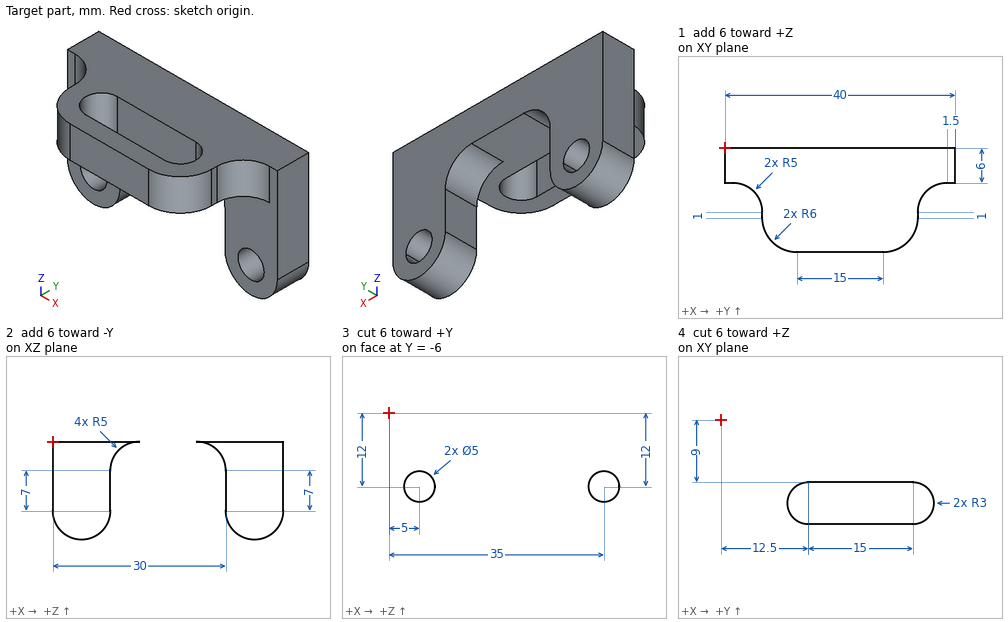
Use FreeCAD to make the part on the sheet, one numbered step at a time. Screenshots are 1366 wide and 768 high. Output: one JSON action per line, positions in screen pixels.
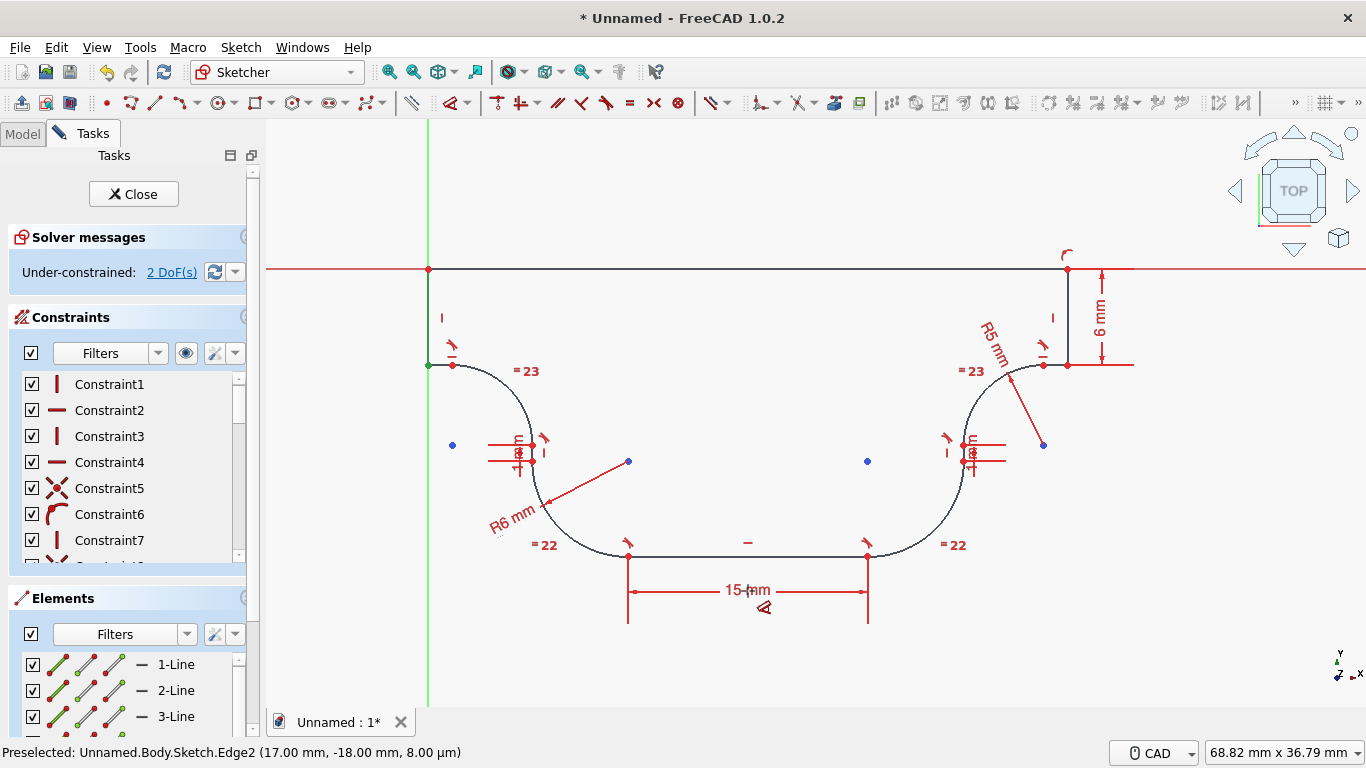
{"action": "left_click", "coordinate": [876, 269]}
{"action": "left_click", "coordinate": [748, 235]}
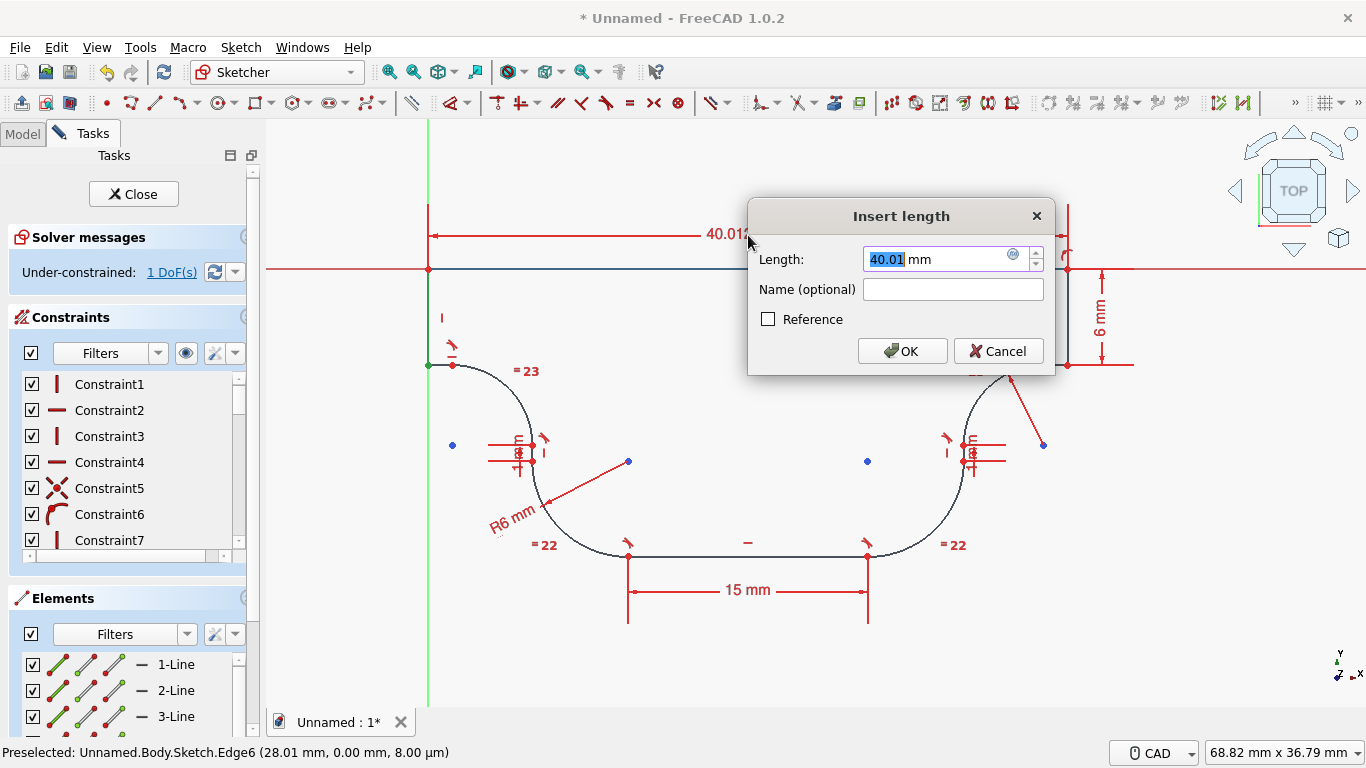
{"action": "type", "text": "40"}
{"action": "key", "text": "Return"}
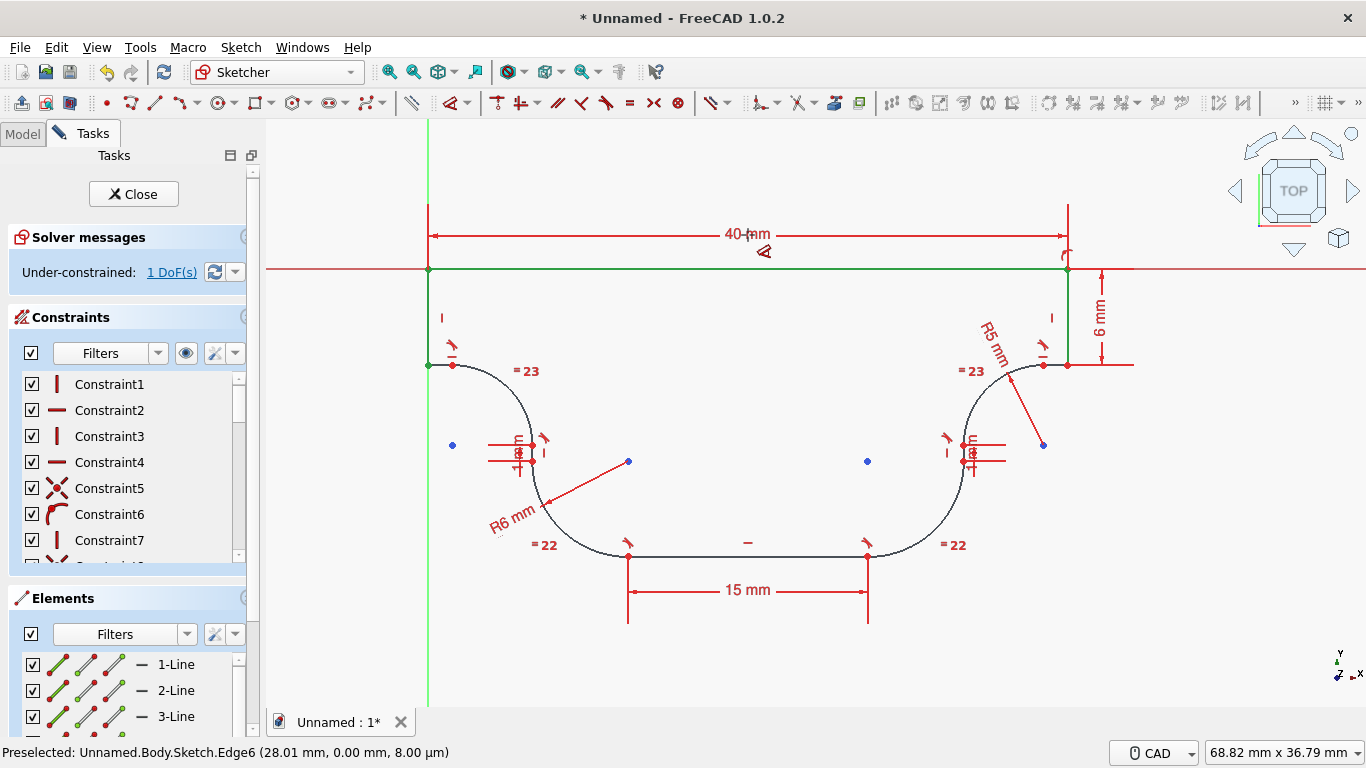
{"action": "scroll", "coordinate": [1053, 365], "scroll_direction": "up", "scroll_amount": 3}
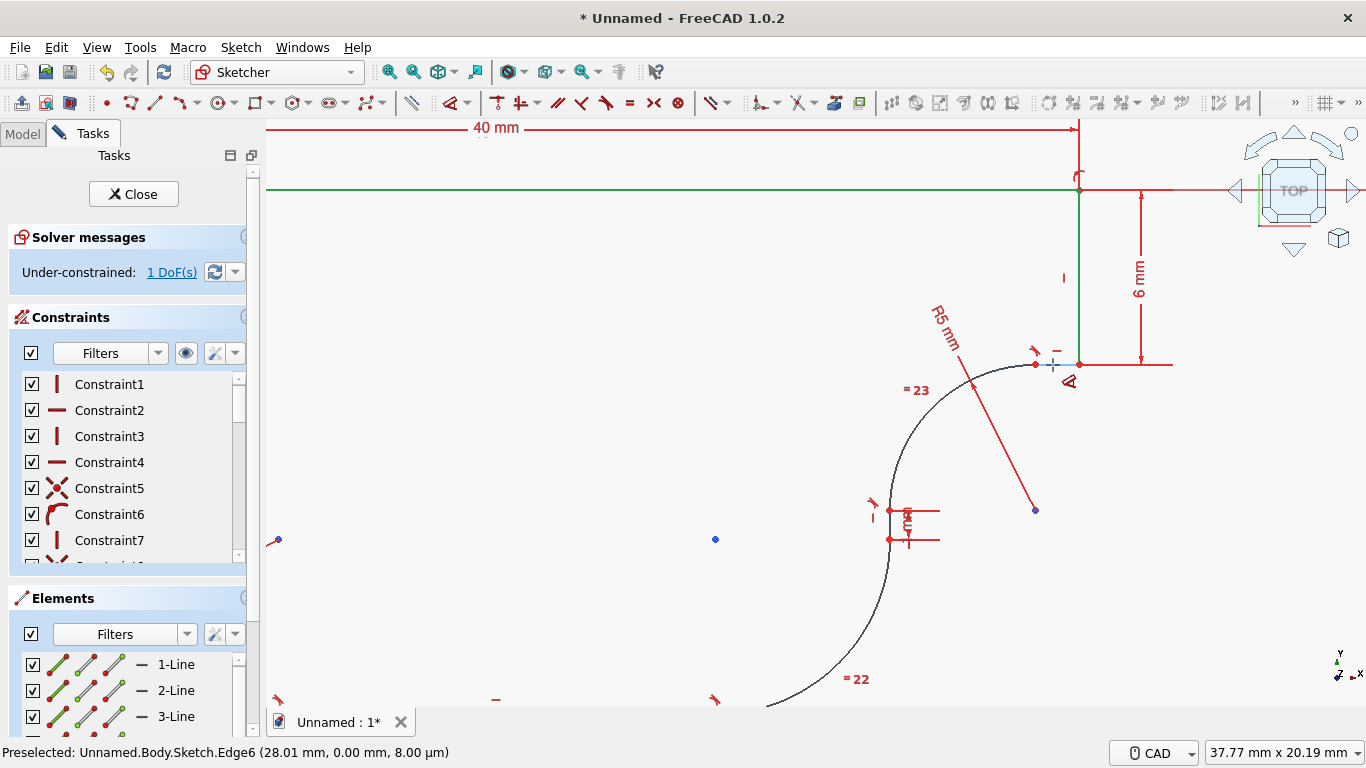
{"action": "left_click", "coordinate": [1053, 365]}
{"action": "left_click", "coordinate": [1057, 331]}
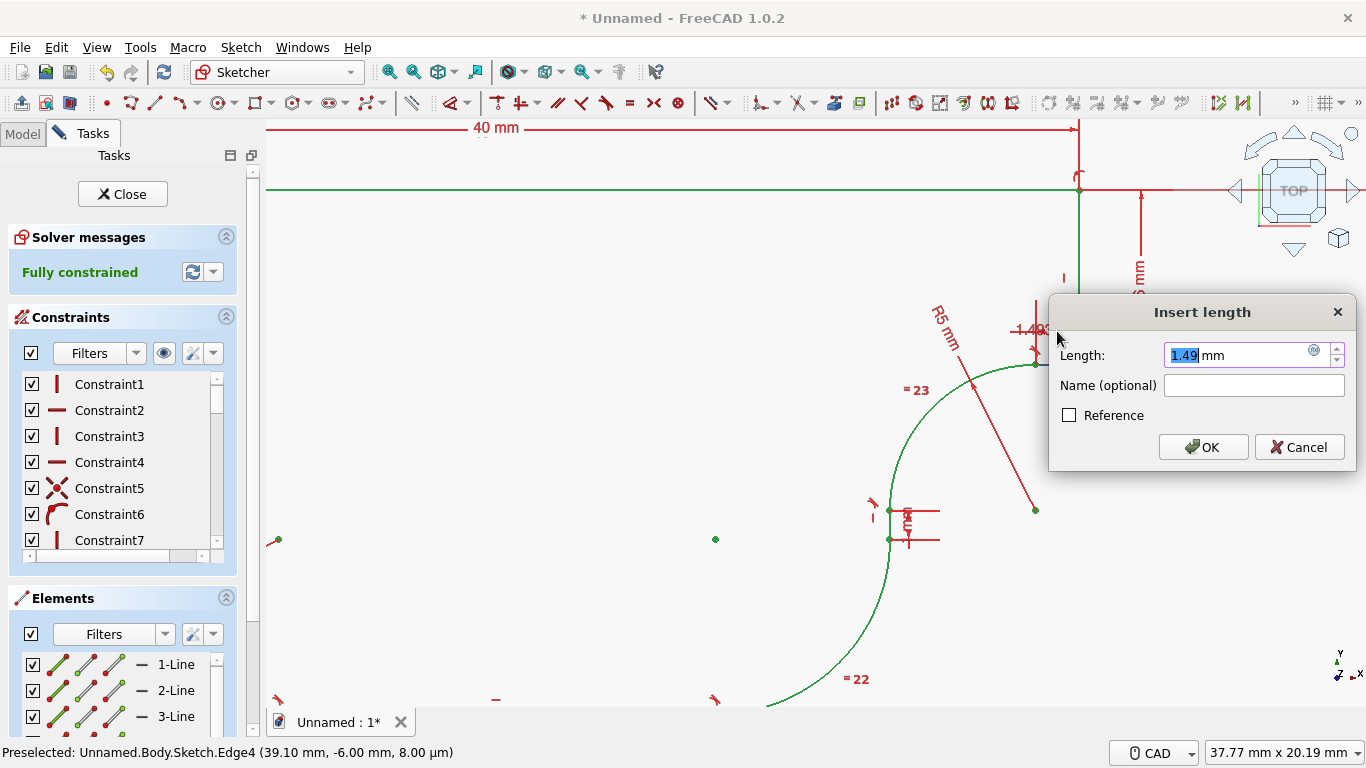
{"action": "type", "text": "1.5"}
{"action": "key", "text": "Return"}
{"action": "key", "text": "Escape"}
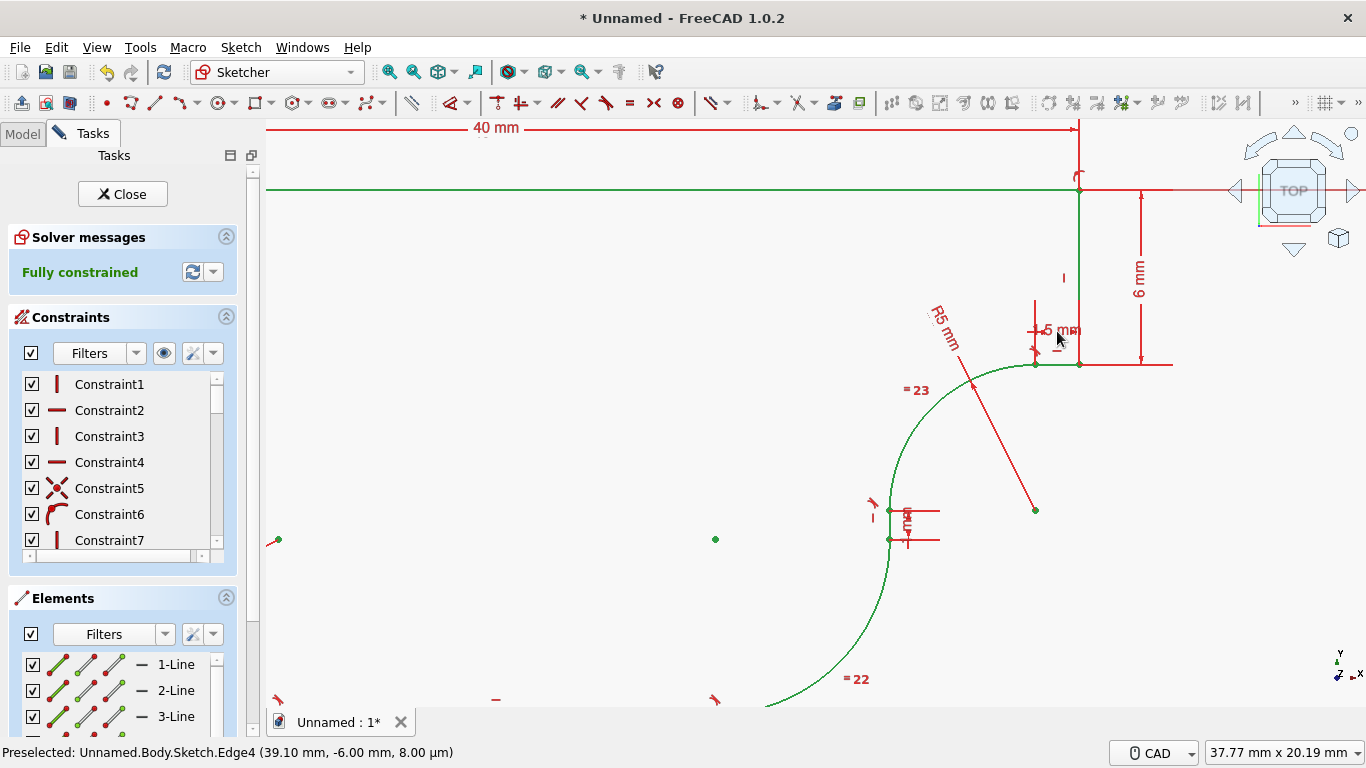
{"action": "left_click", "coordinate": [123, 194]}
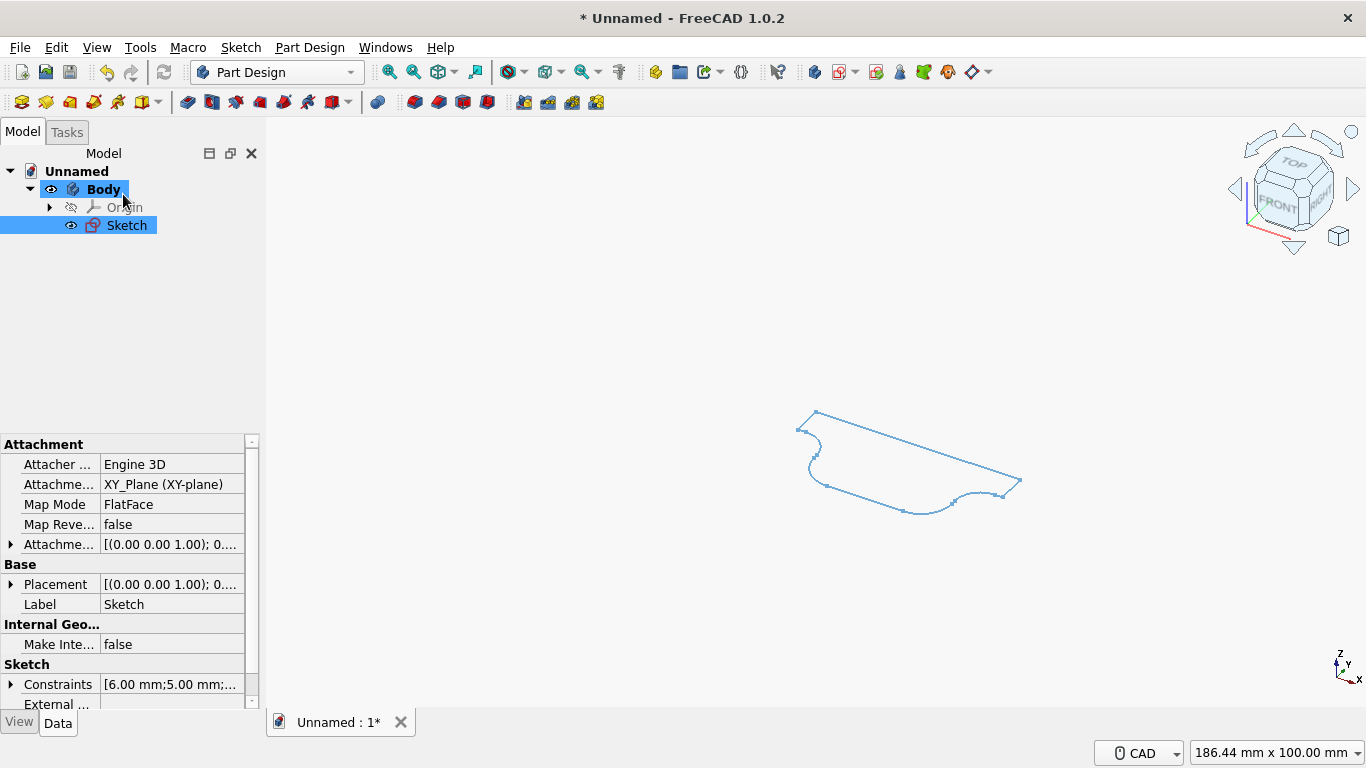
{"action": "left_click", "coordinate": [22, 102]}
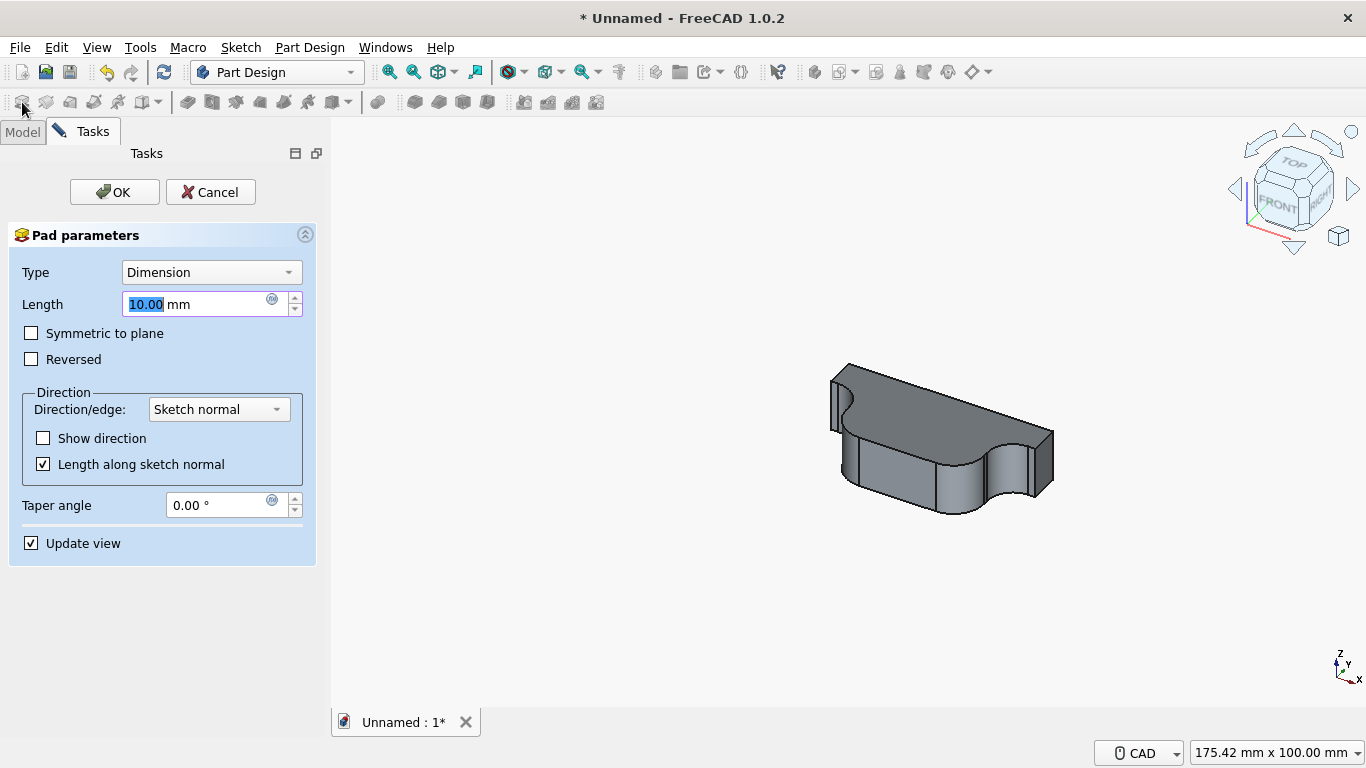
{"action": "type", "text": "6"}
{"action": "key", "text": "Tab"}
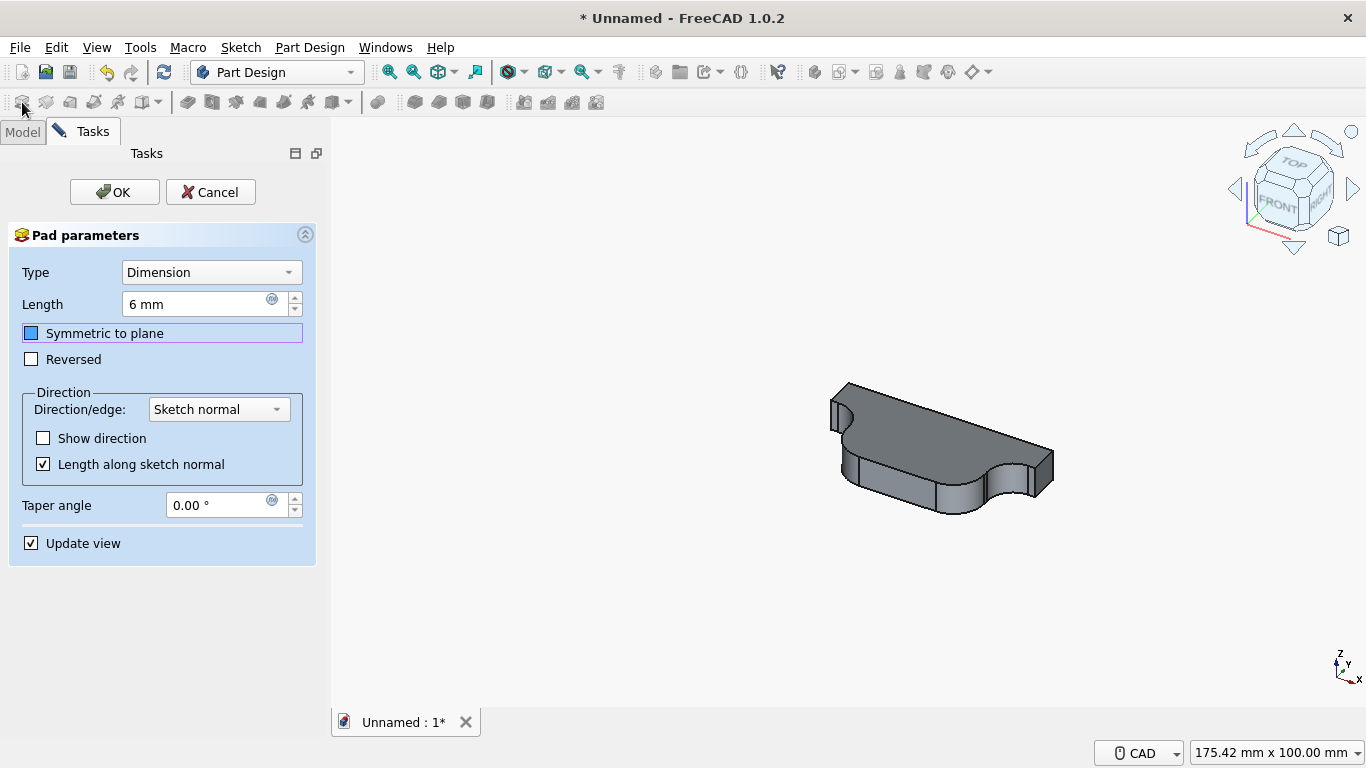
{"action": "left_click", "coordinate": [115, 192]}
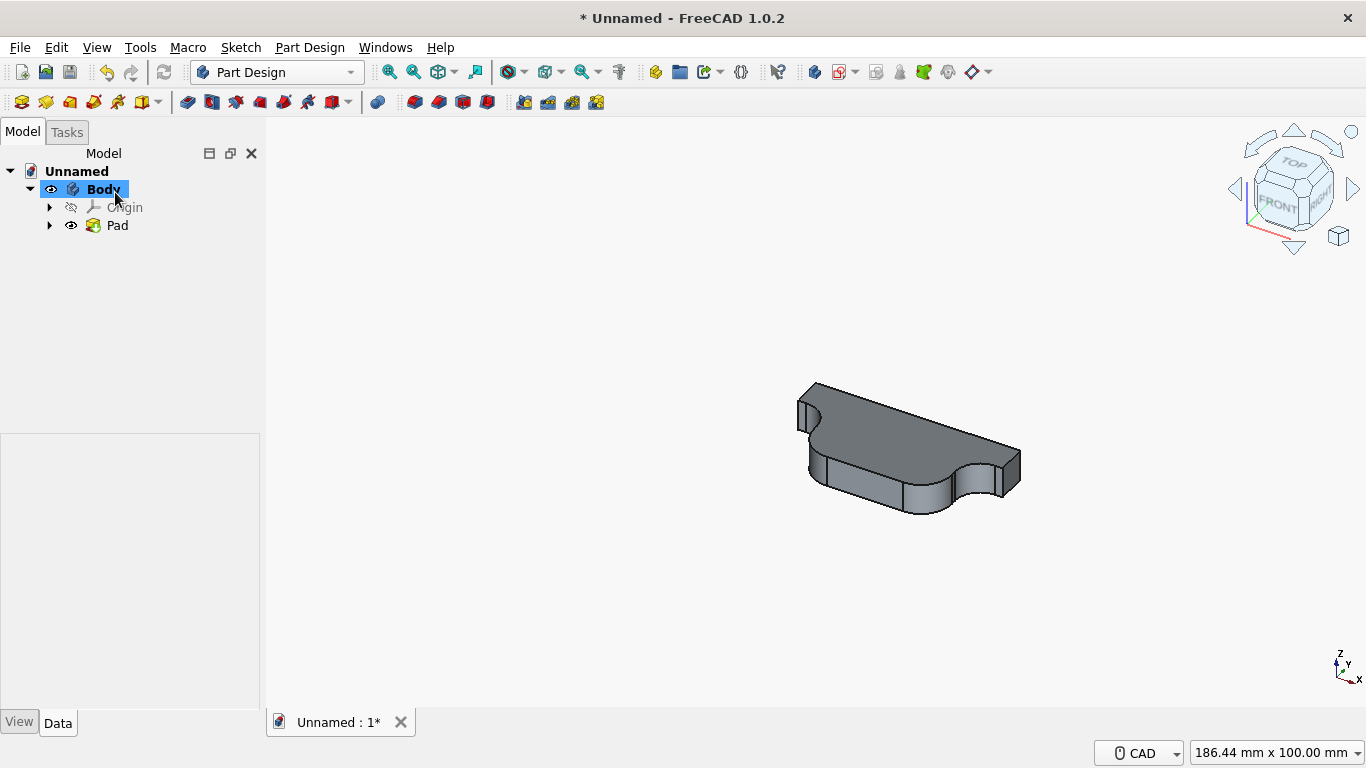
{"action": "key", "text": "v f"}